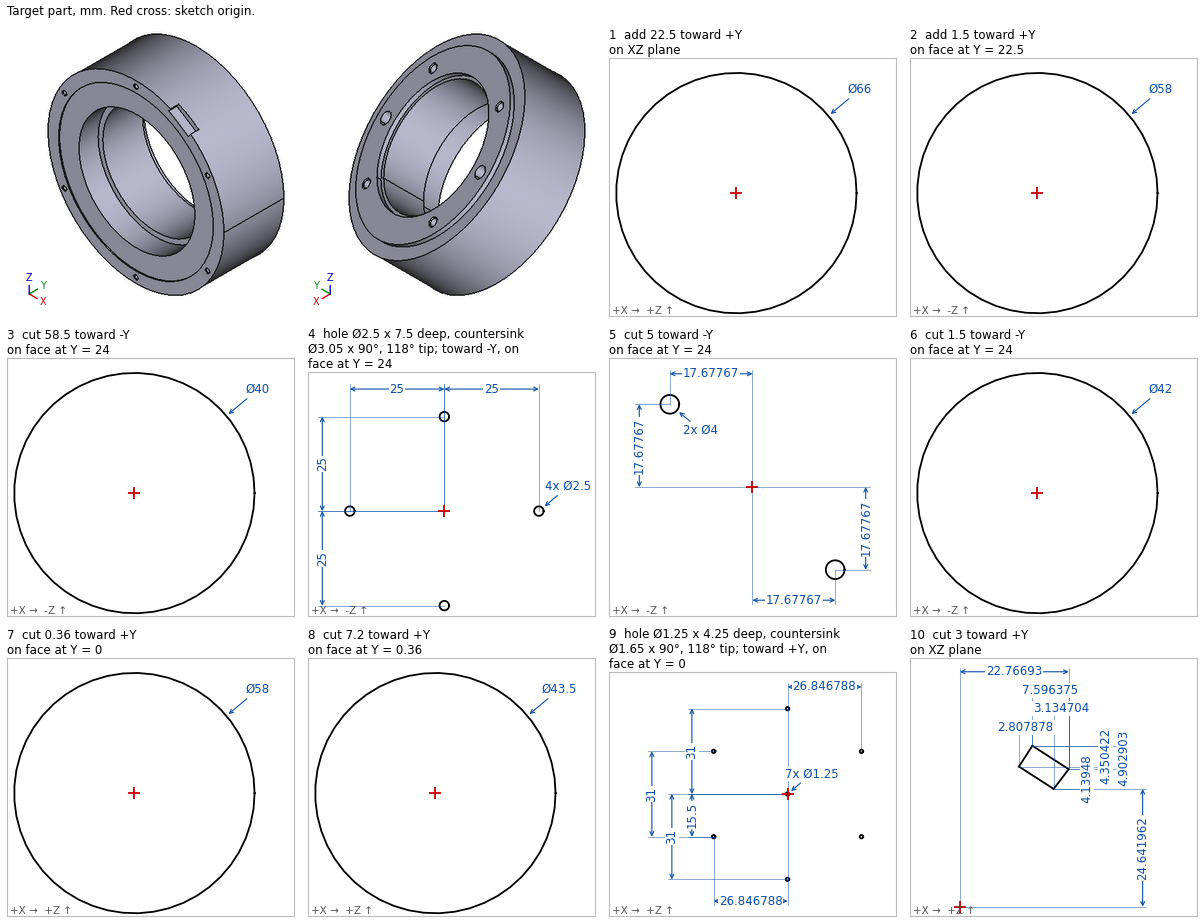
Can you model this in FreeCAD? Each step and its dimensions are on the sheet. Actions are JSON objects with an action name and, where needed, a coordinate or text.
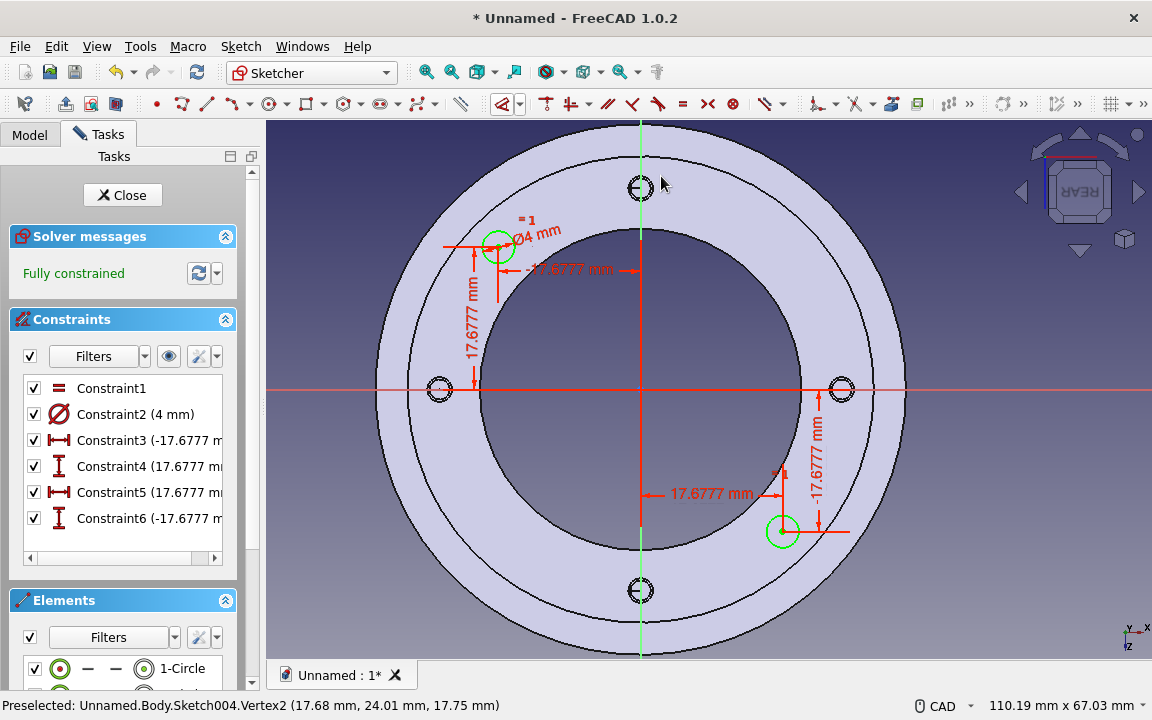
{"action": "left_click", "coordinate": [123, 195]}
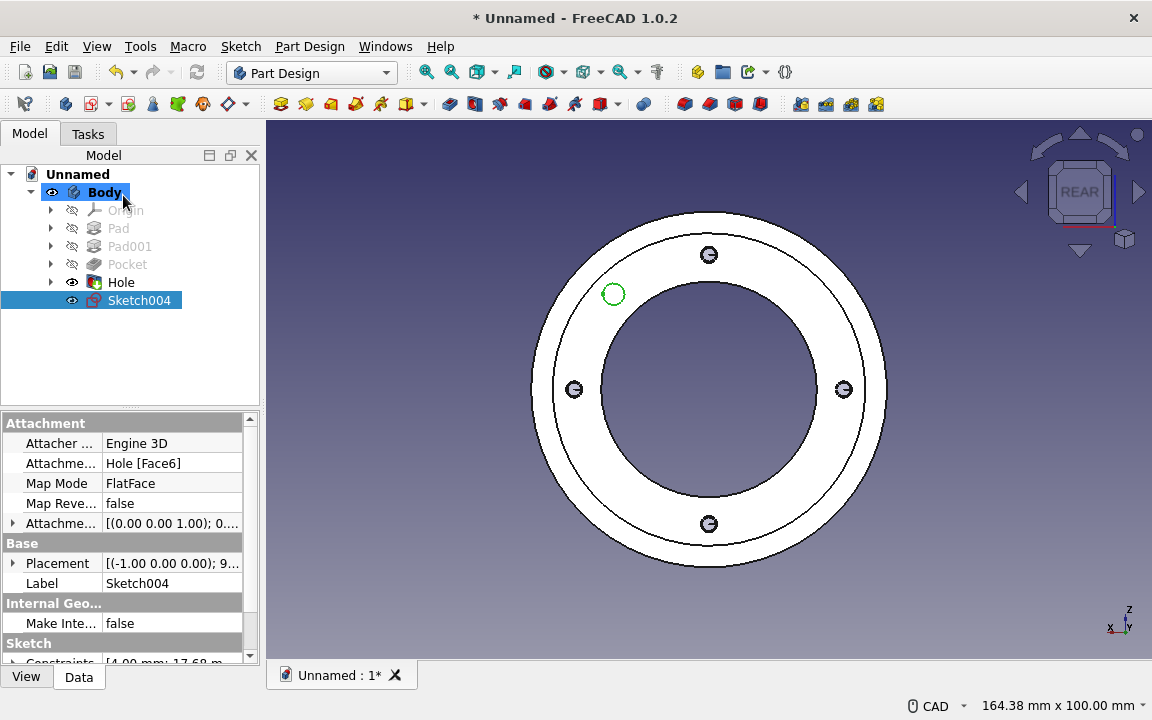
{"action": "left_click", "coordinate": [450, 104]}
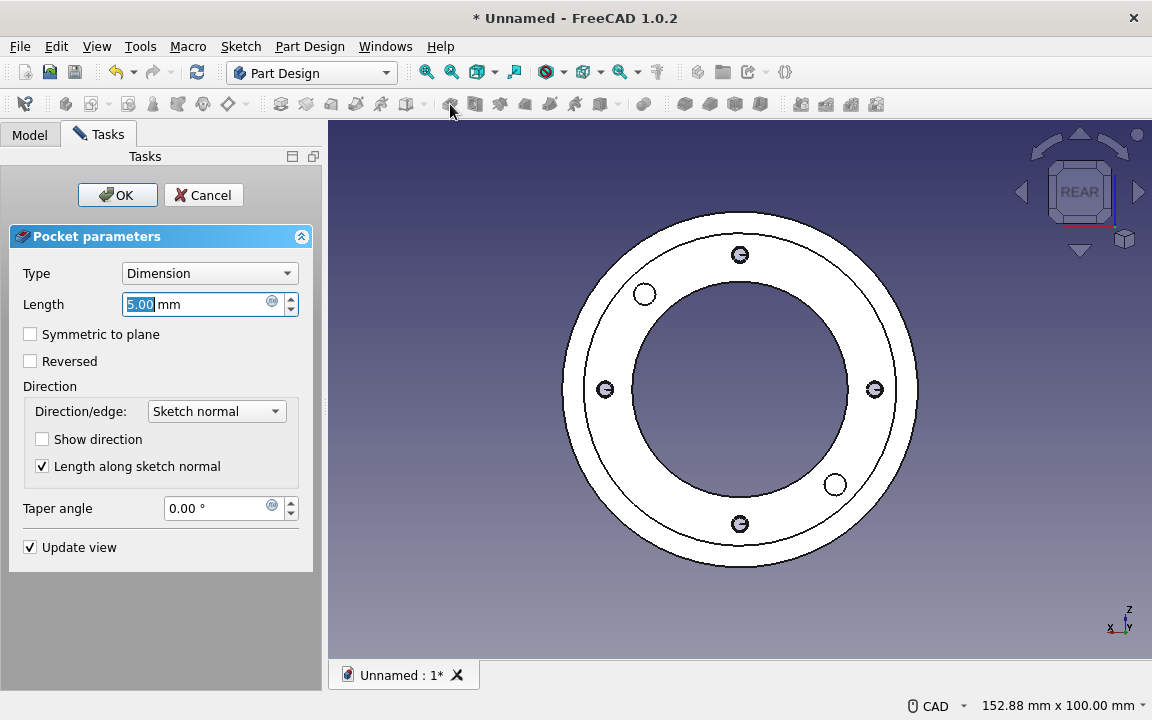
{"action": "type", "text": "5"}
{"action": "key", "text": "Tab"}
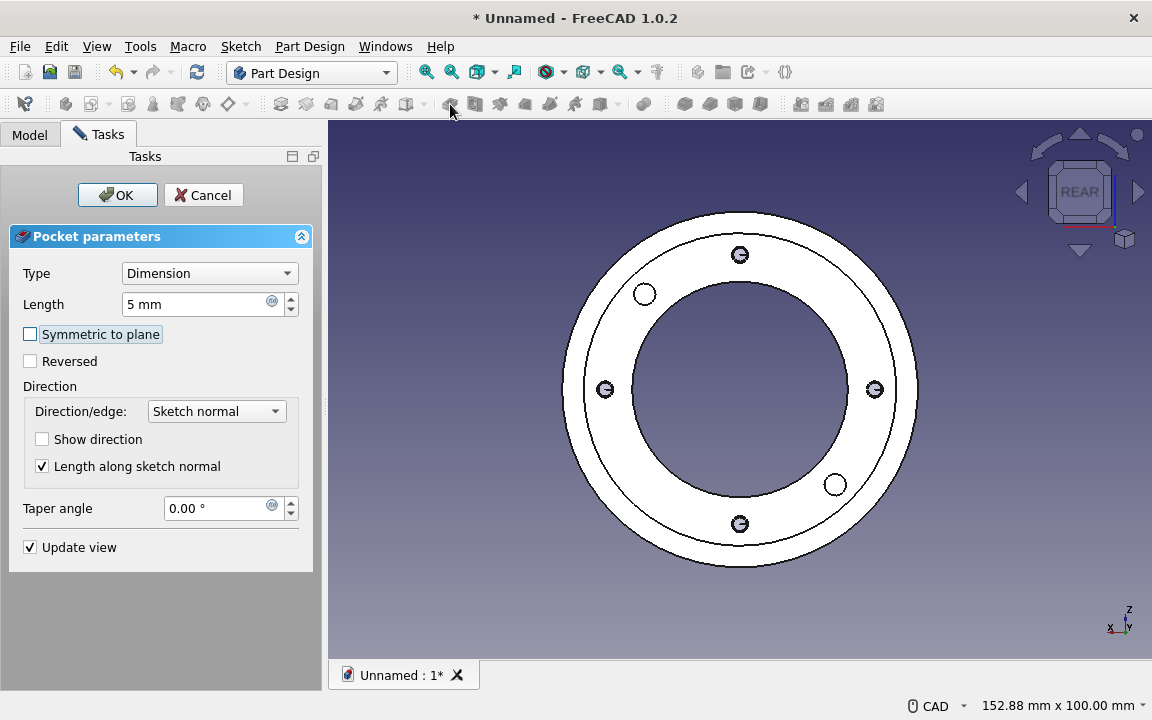
{"action": "left_click", "coordinate": [118, 195]}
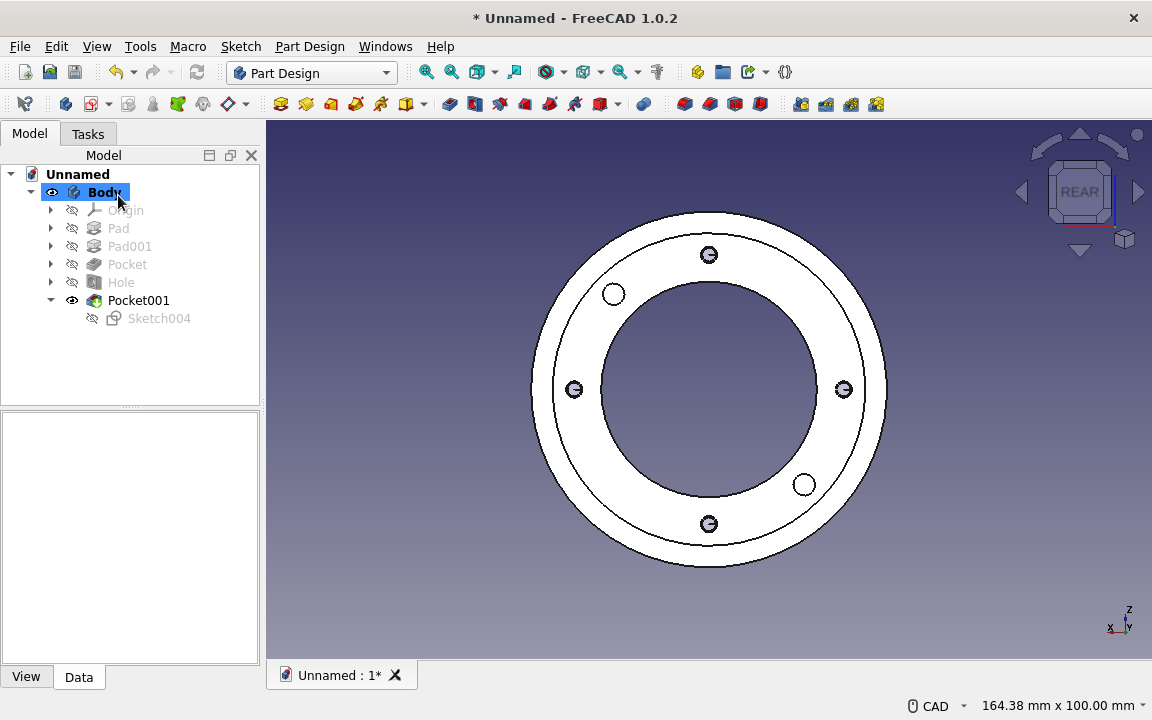
{"action": "left_click", "coordinate": [620, 478]}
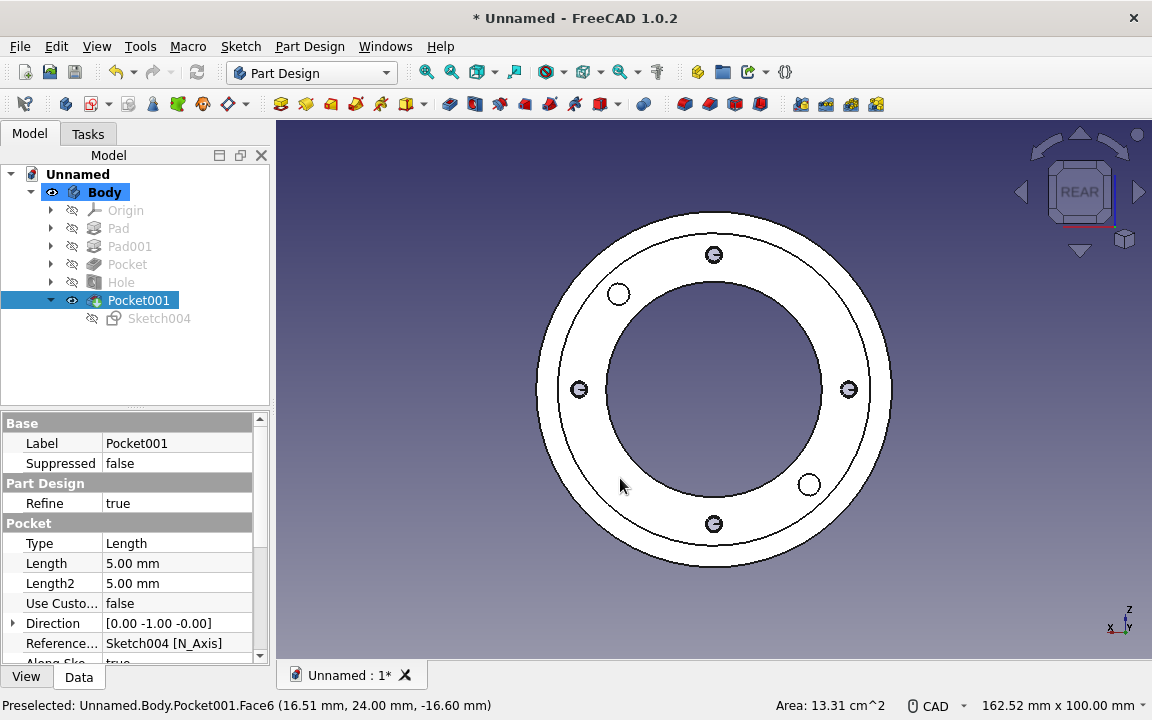
{"action": "left_click", "coordinate": [90, 104]}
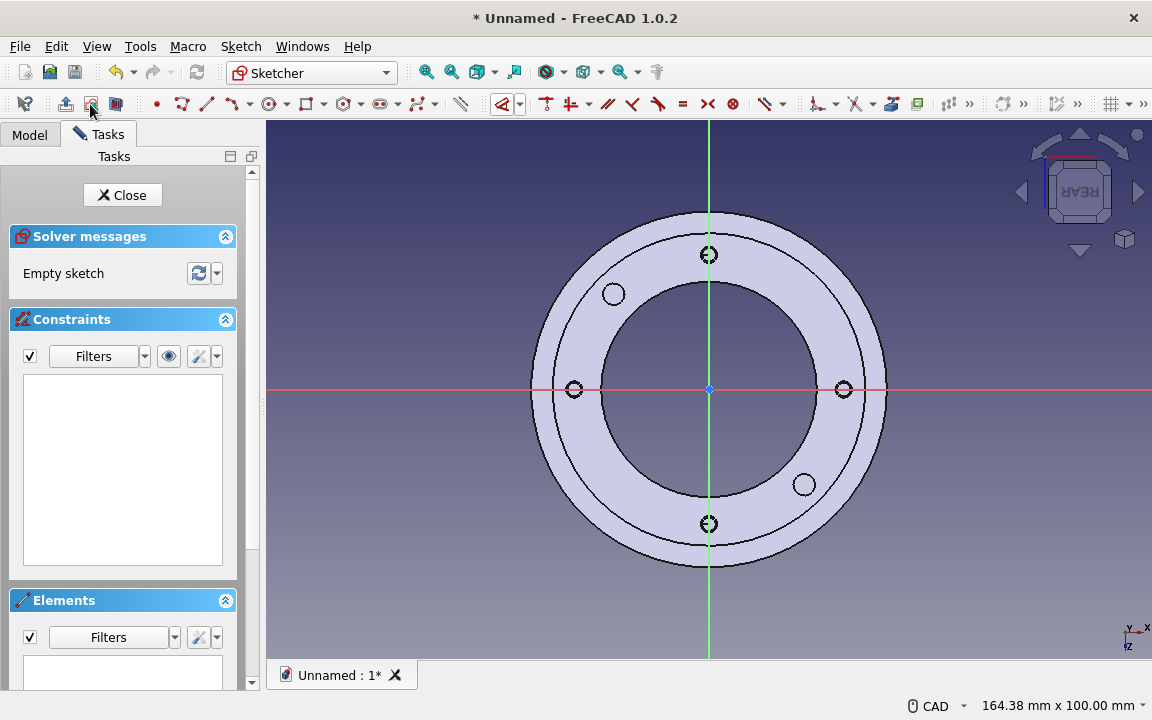
{"action": "scroll", "coordinate": [848, 389], "scroll_direction": "up", "scroll_amount": 2}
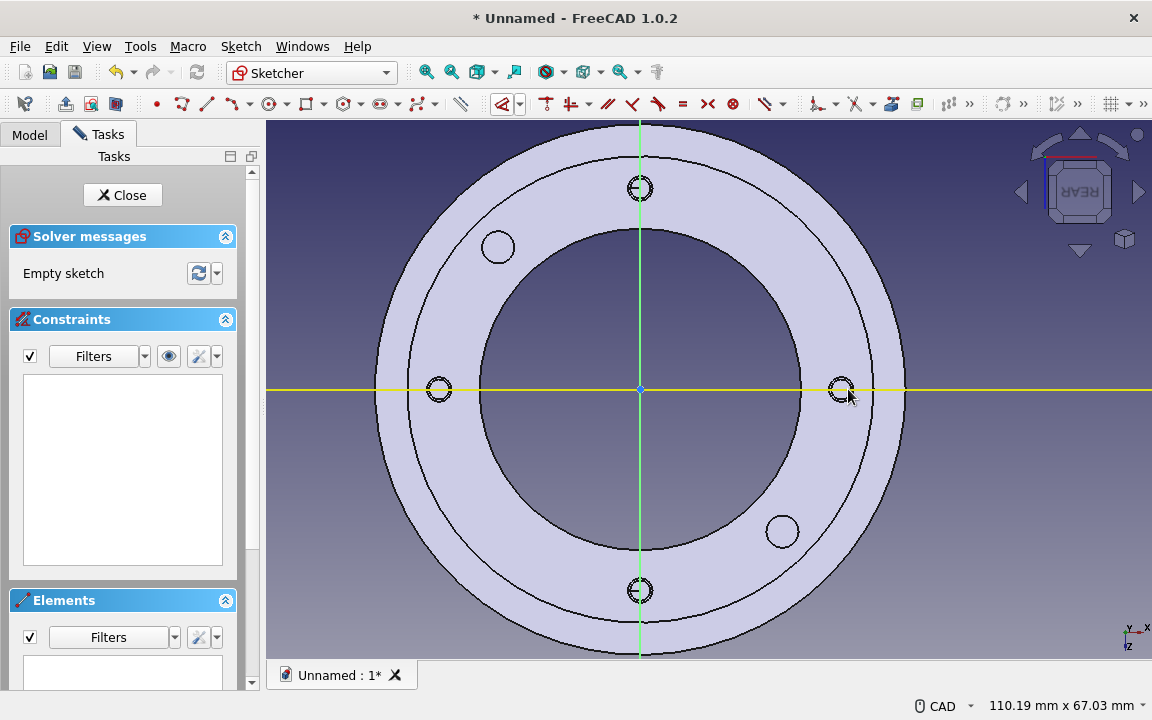
{"action": "left_click", "coordinate": [268, 104]}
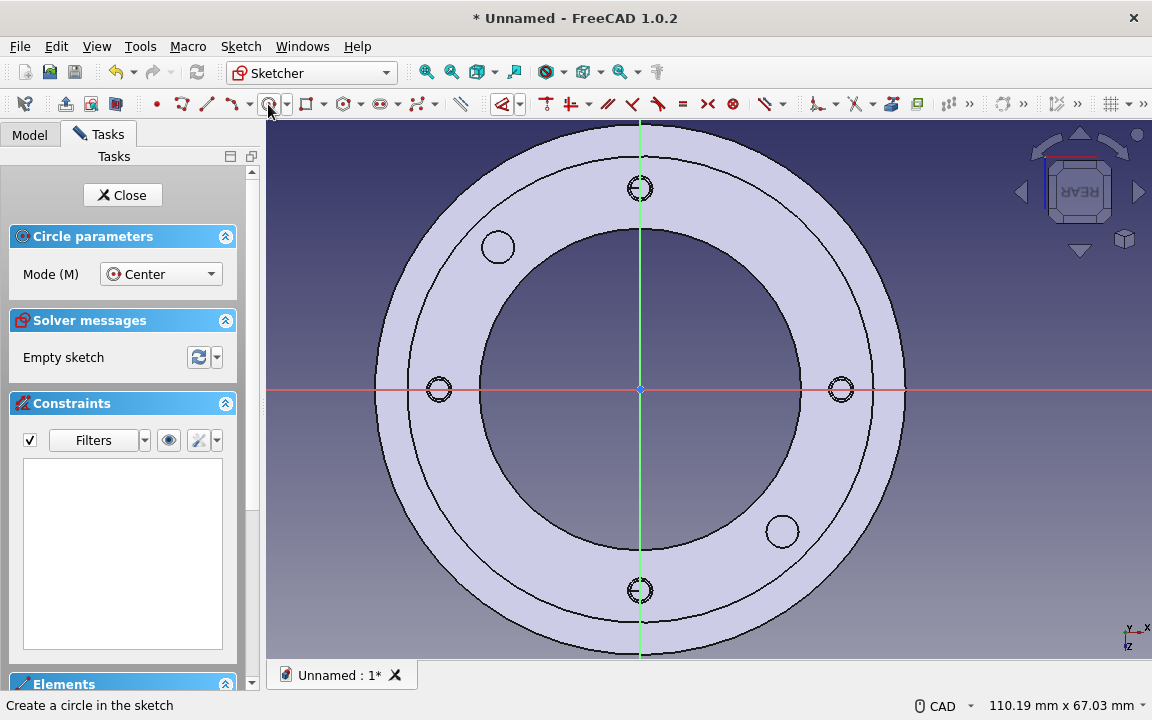
{"action": "left_click", "coordinate": [640, 389]}
{"action": "left_click", "coordinate": [760, 270]}
{"action": "key", "text": "Escape"}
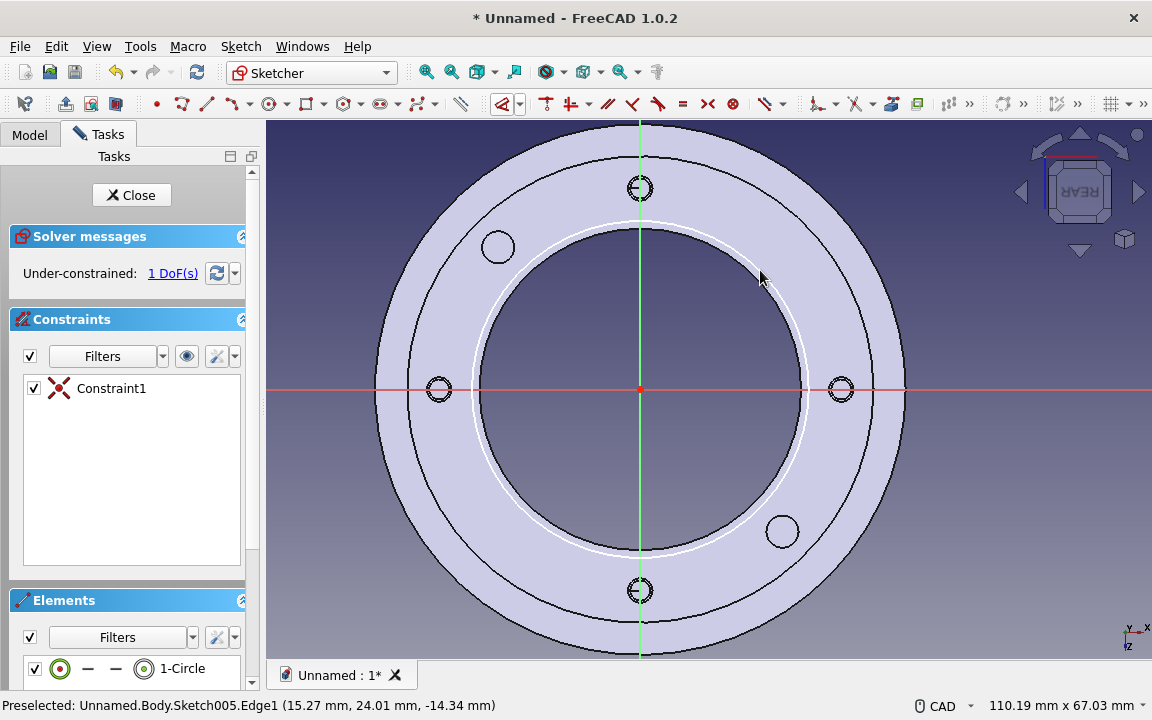
{"action": "left_click", "coordinate": [759, 270]}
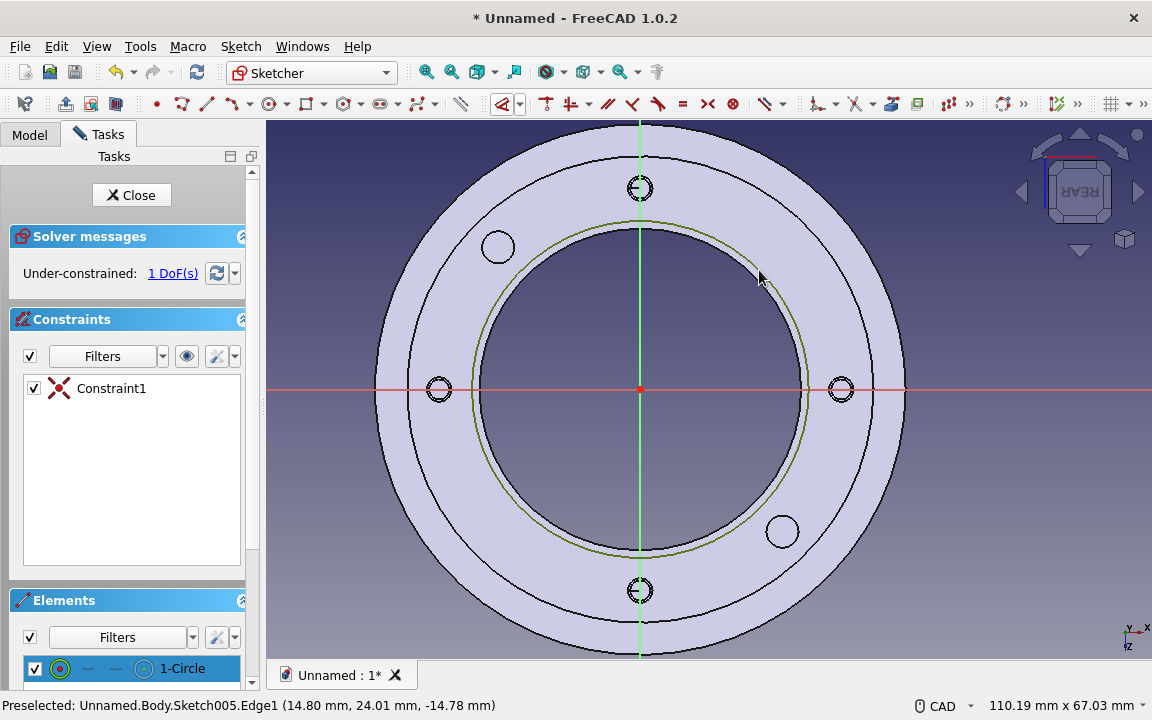
{"action": "key", "text": "k o"}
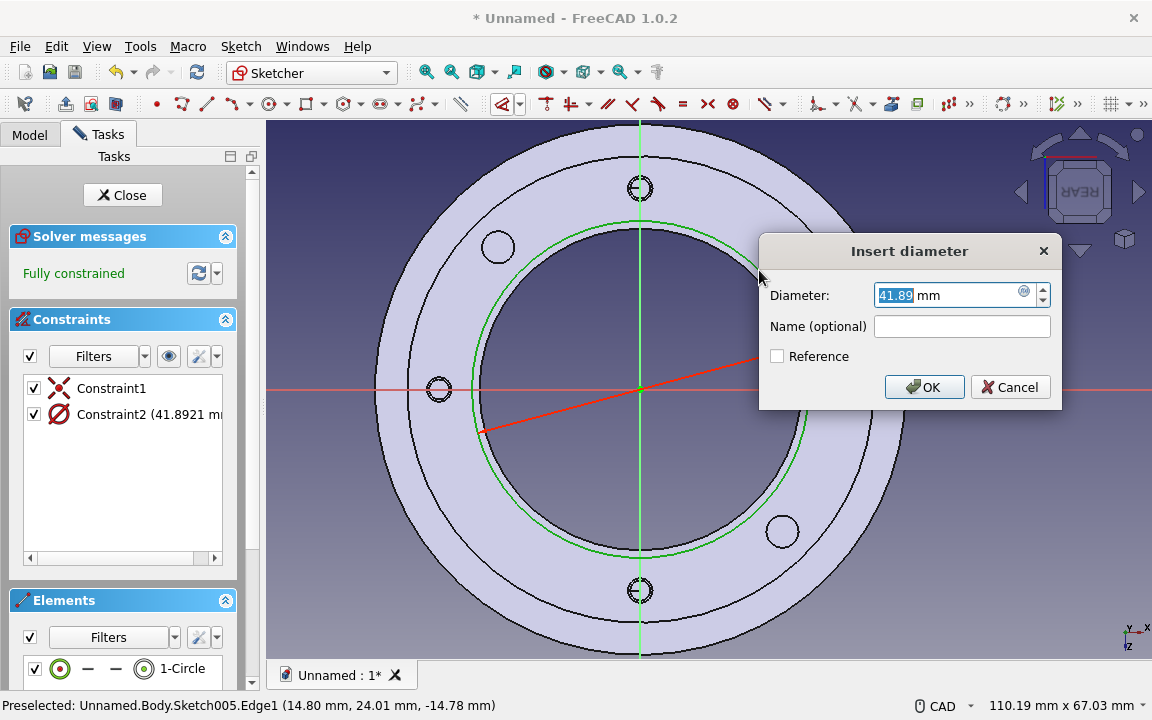
{"action": "type", "text": "42"}
{"action": "key", "text": "Return"}